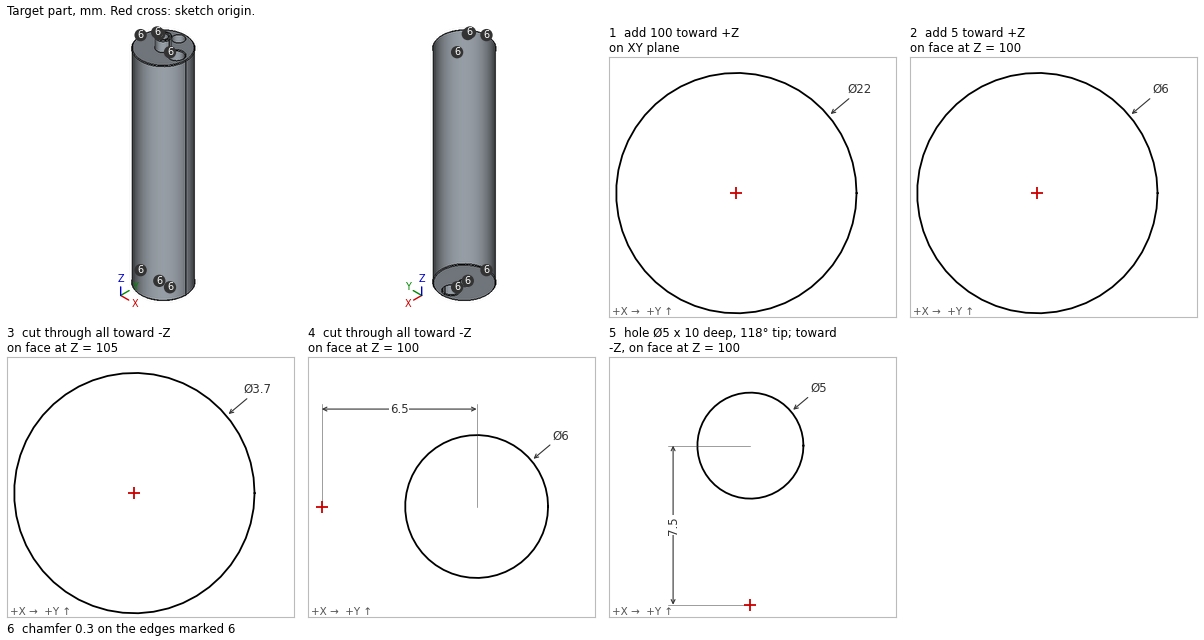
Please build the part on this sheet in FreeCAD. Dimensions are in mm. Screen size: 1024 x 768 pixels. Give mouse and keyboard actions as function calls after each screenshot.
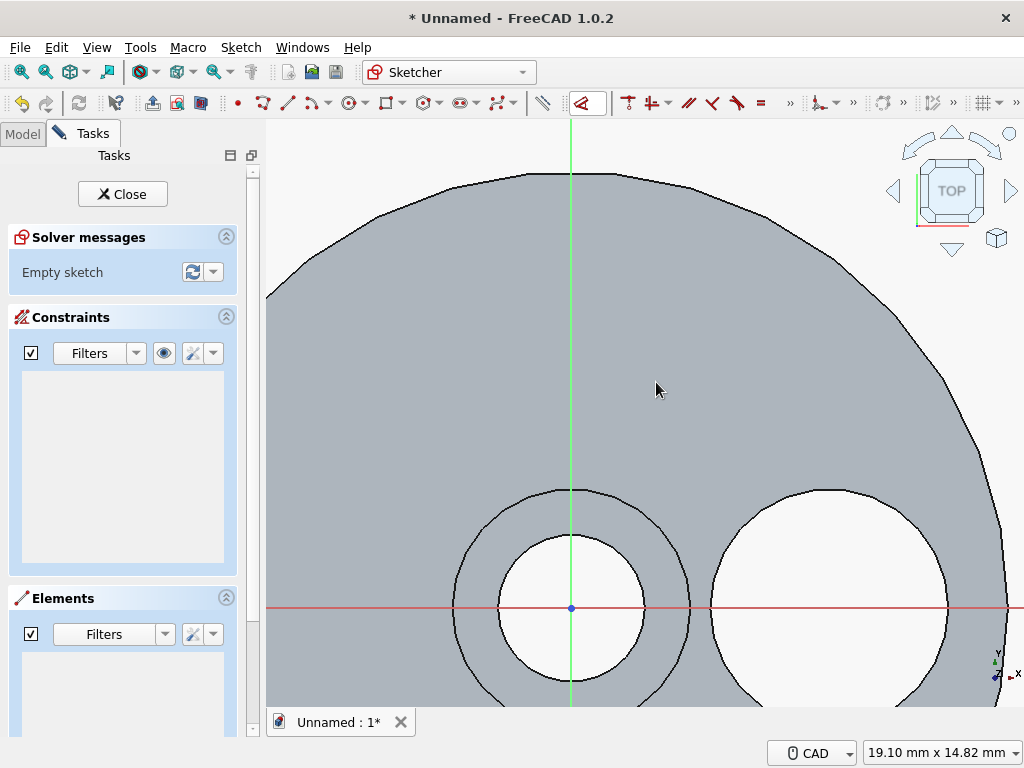
click(350, 104)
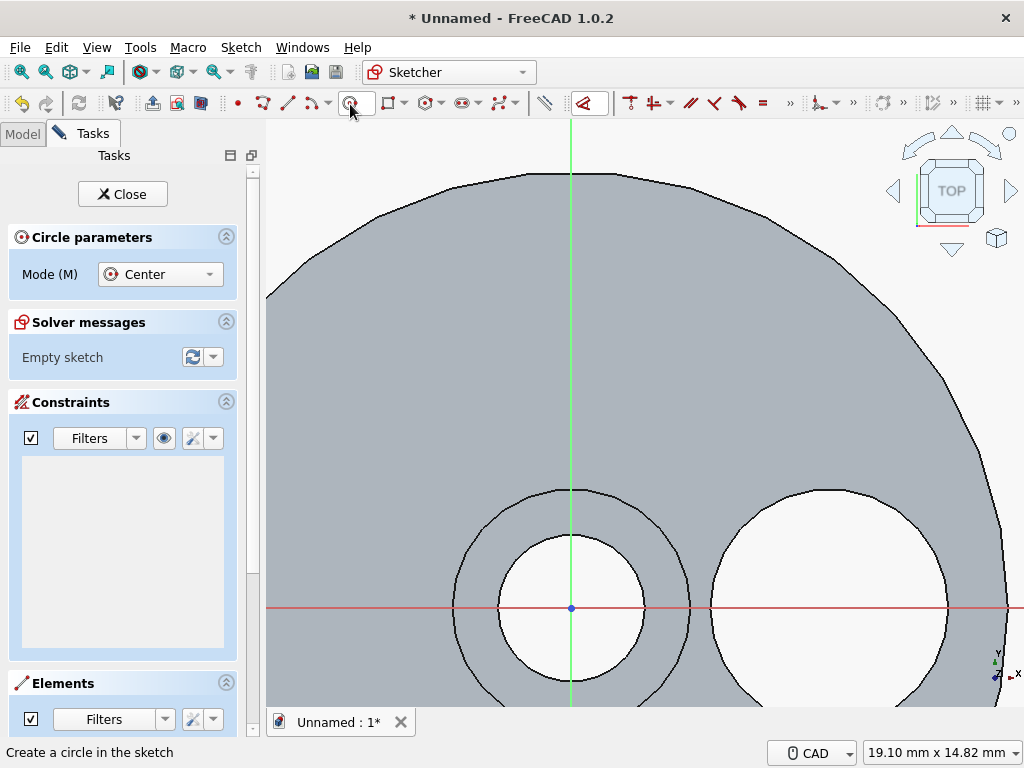
click(571, 311)
click(642, 240)
key(Escape)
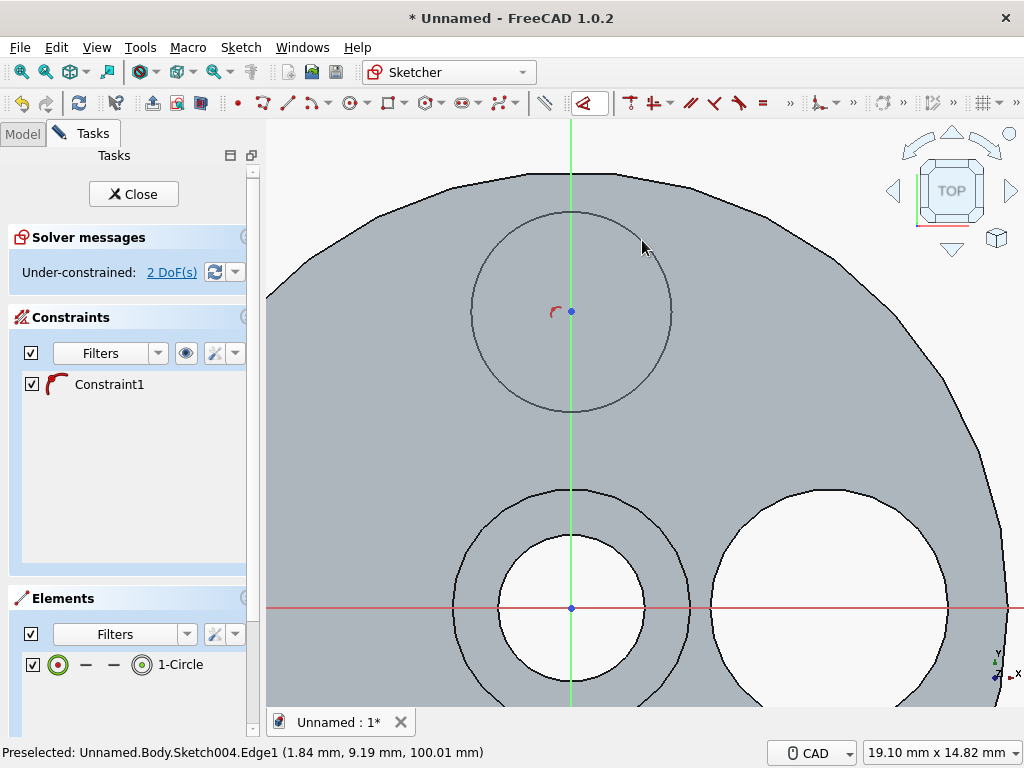
click(642, 241)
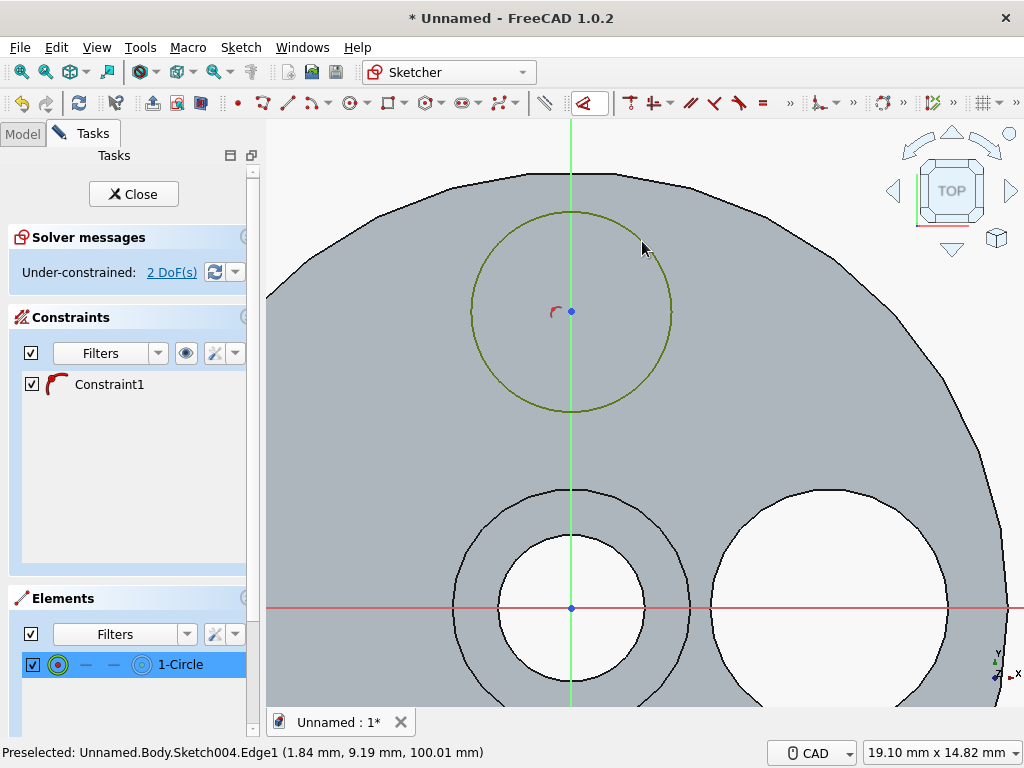
click(602, 104)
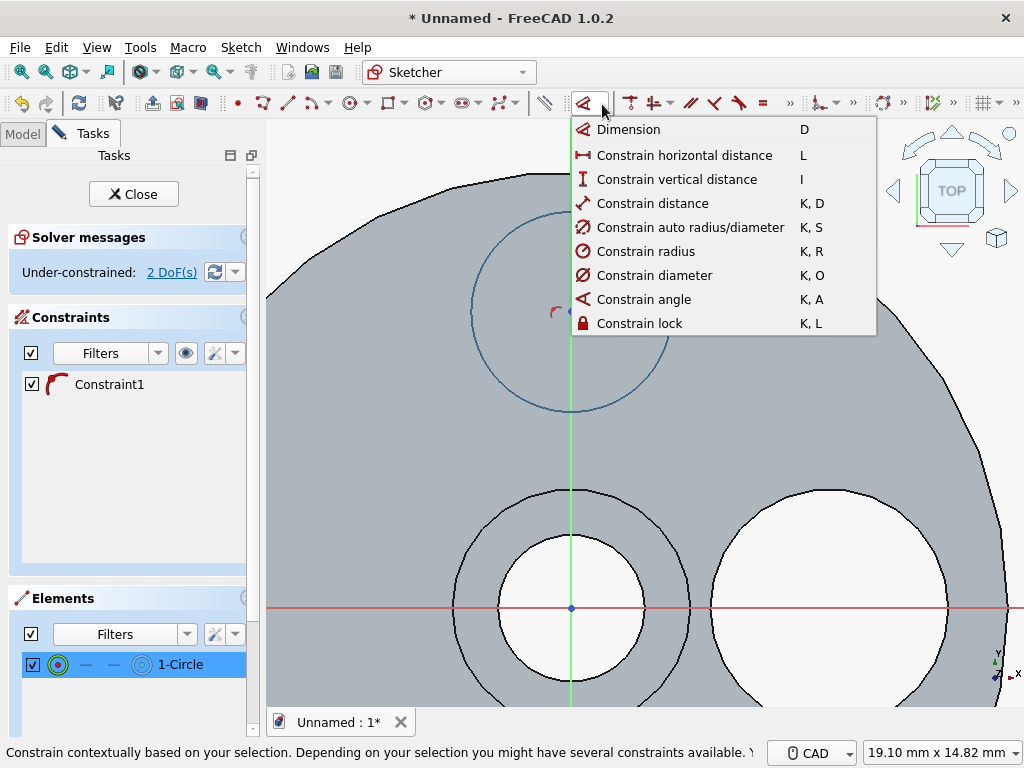
click(724, 275)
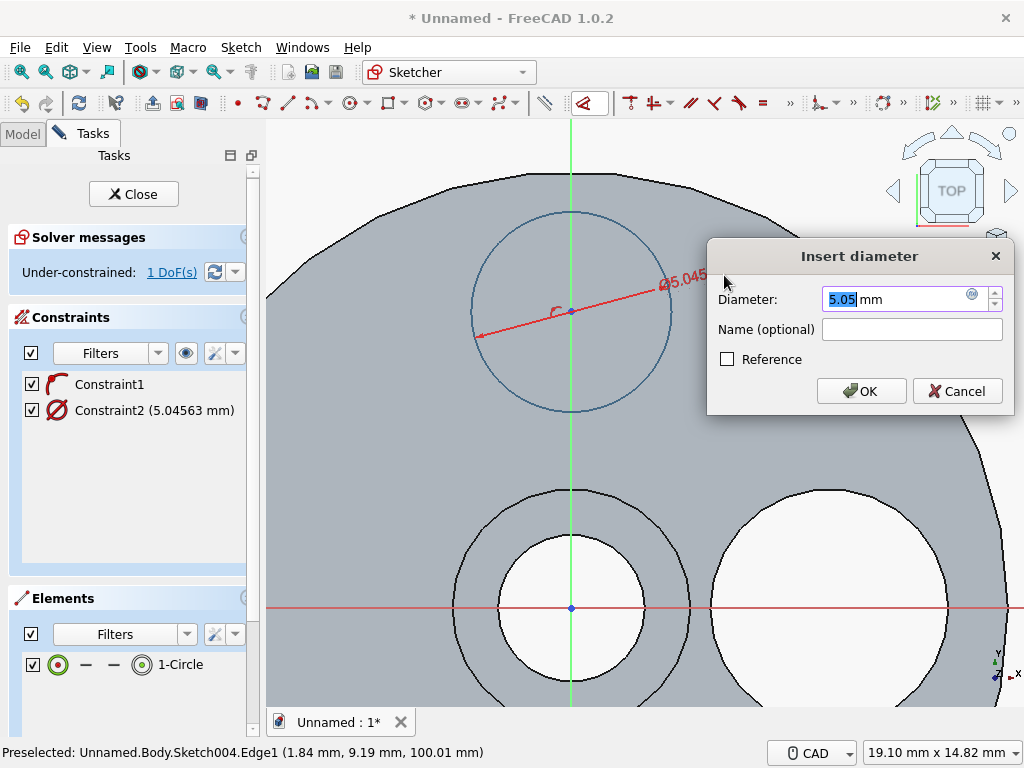
text(5)
key(Return)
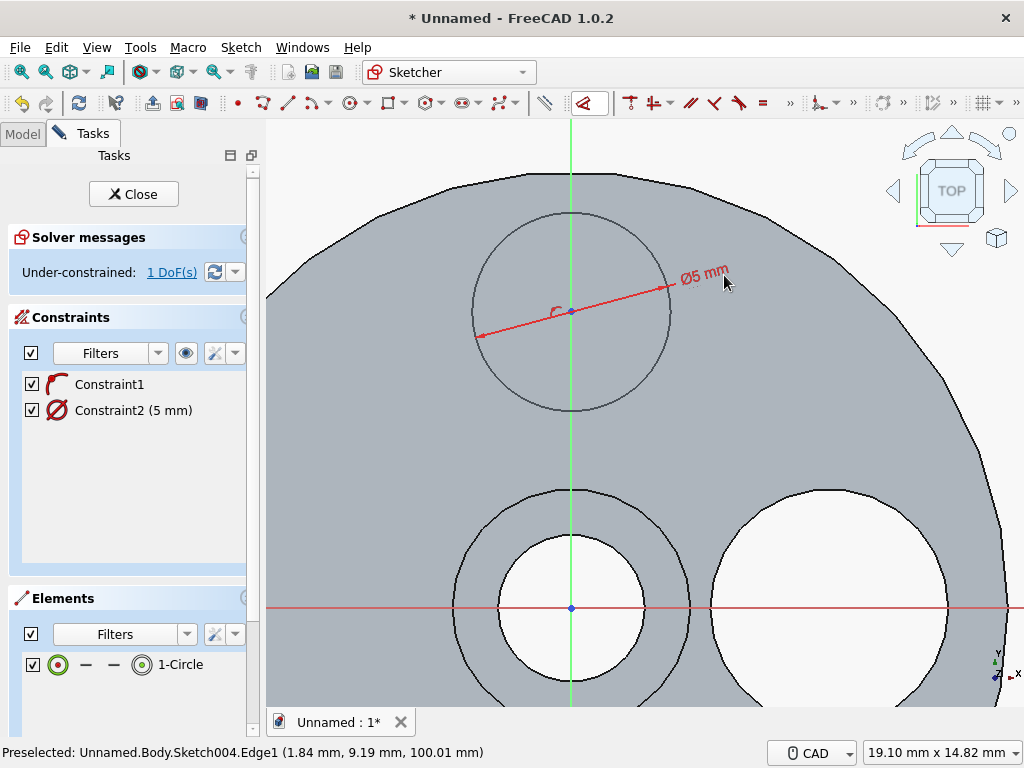
click(571, 312)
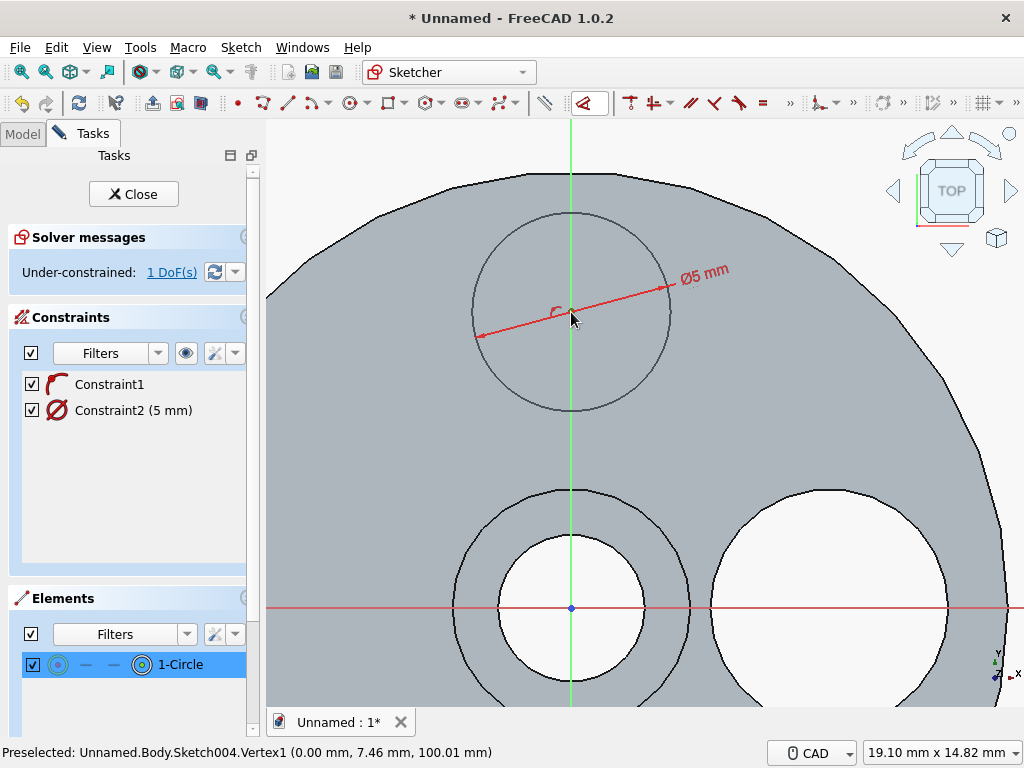
click(602, 104)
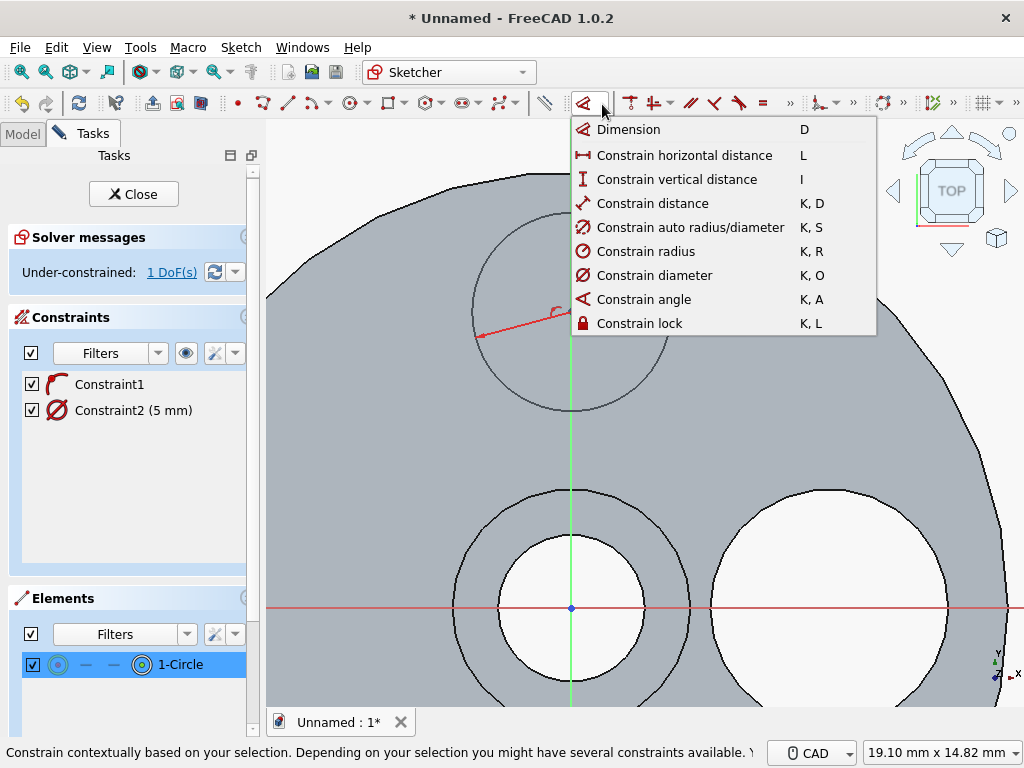
click(724, 179)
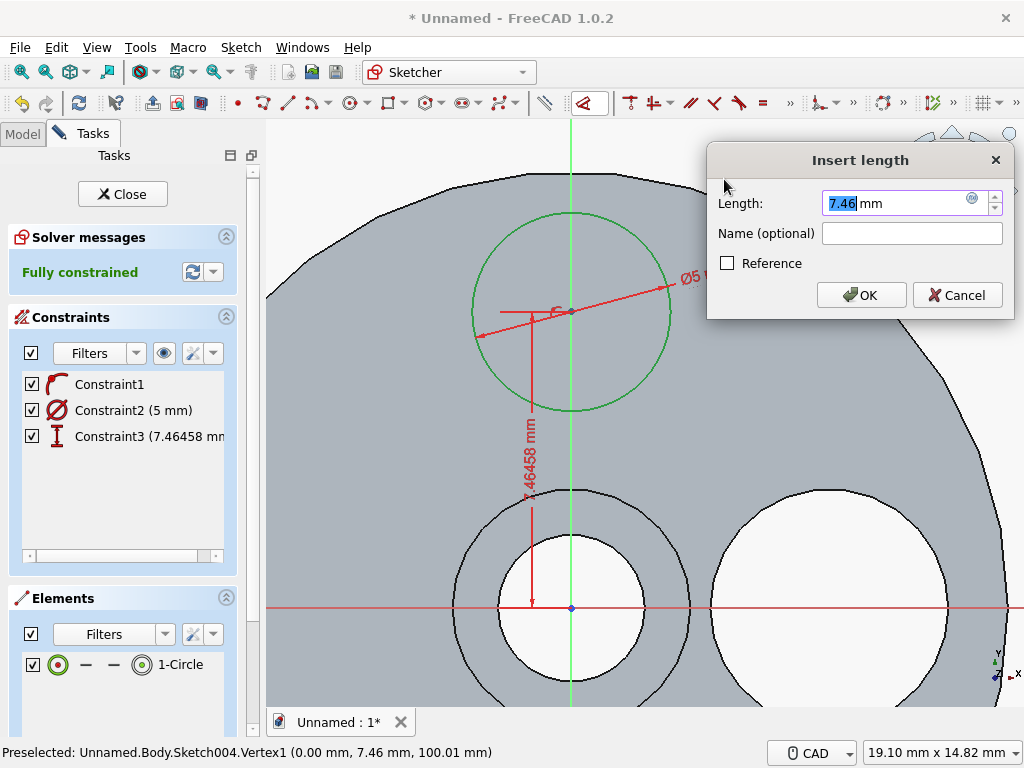
text(7.5)
key(Return)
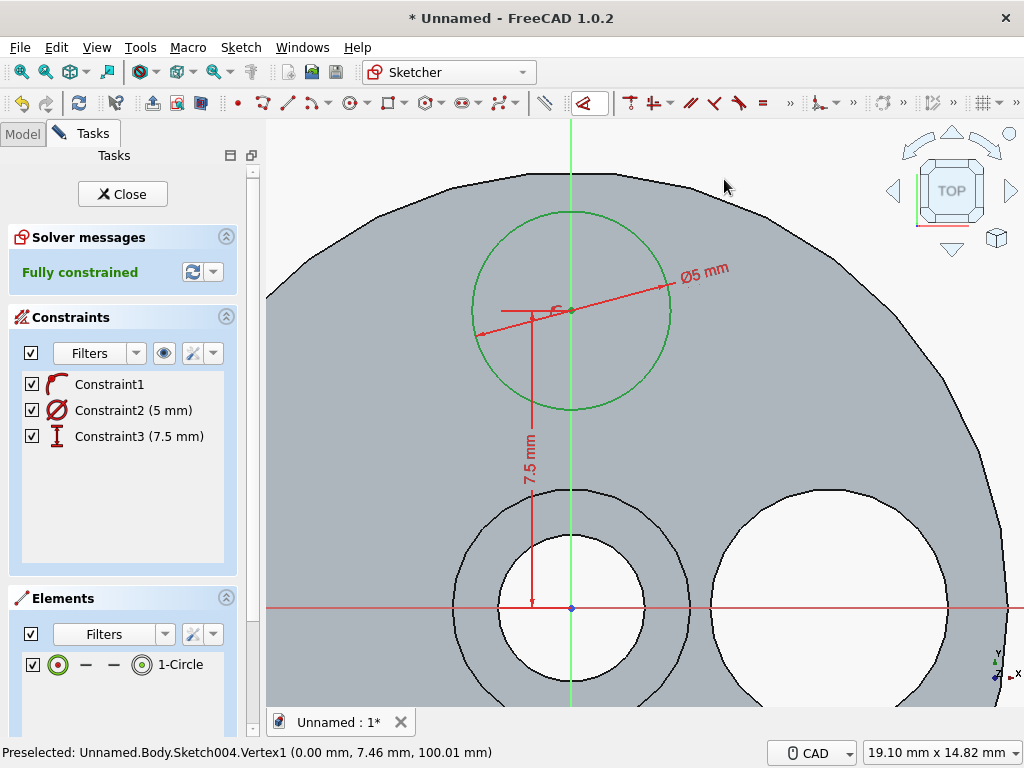
click(123, 194)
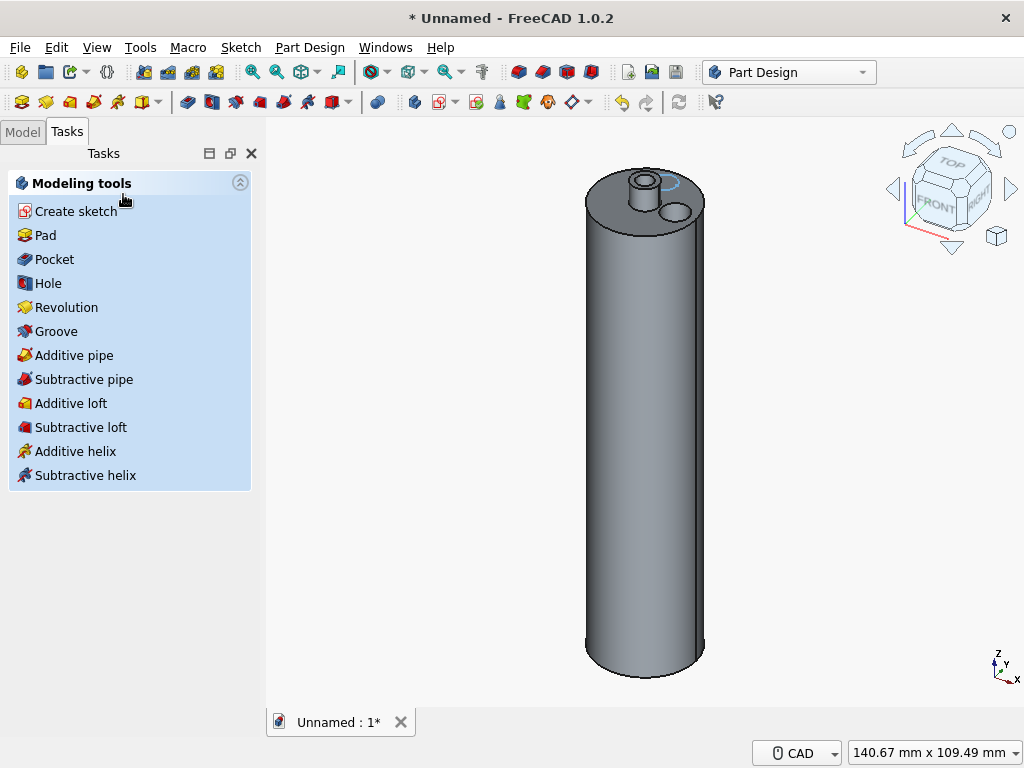
click(212, 102)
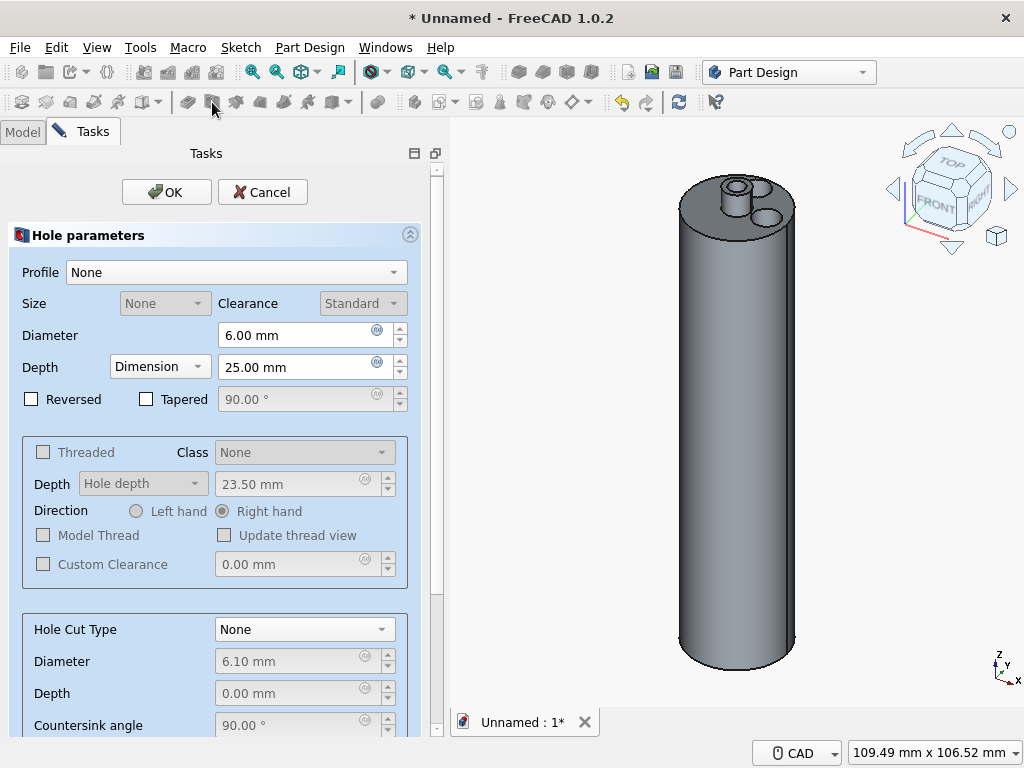
triple_click(305, 335)